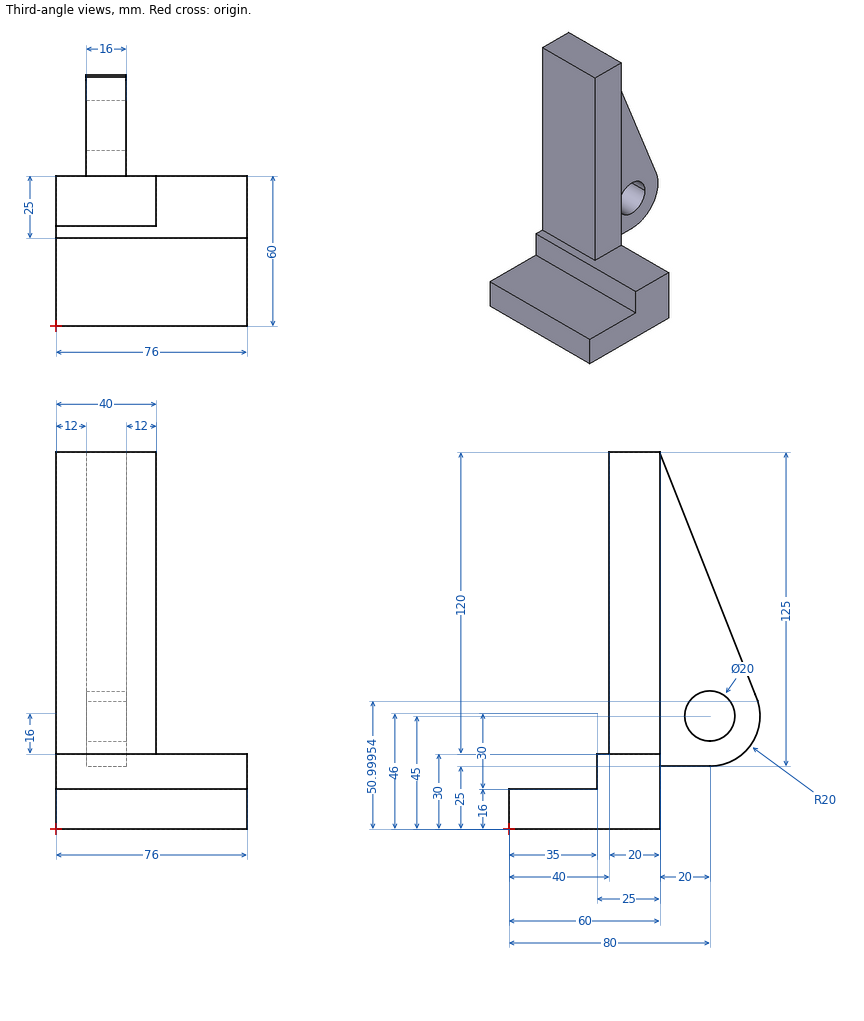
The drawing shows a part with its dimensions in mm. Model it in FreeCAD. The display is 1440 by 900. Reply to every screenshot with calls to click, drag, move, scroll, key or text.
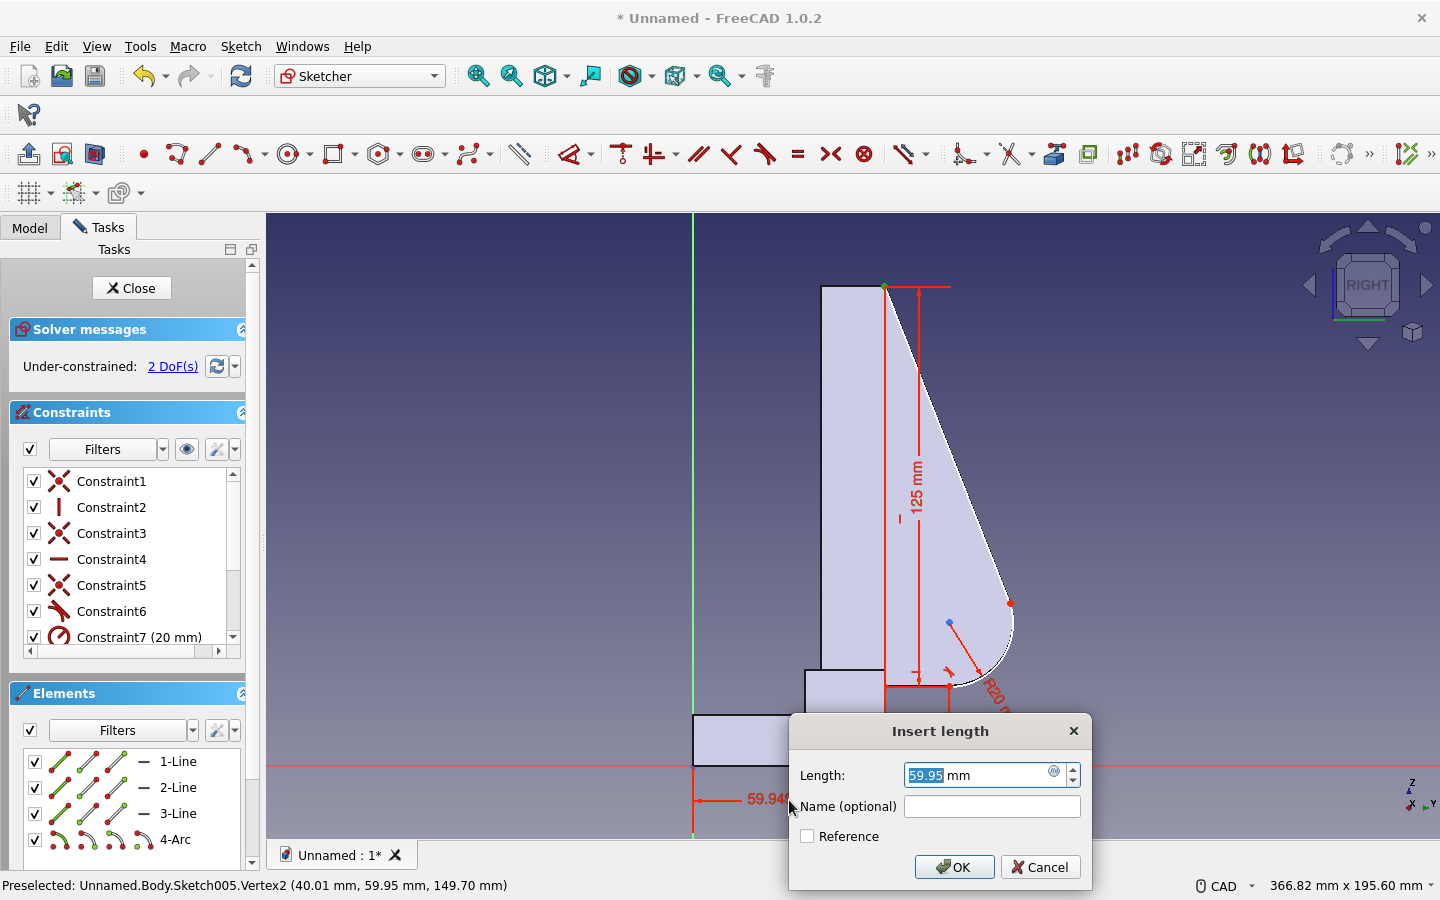
text(60)
key(Return)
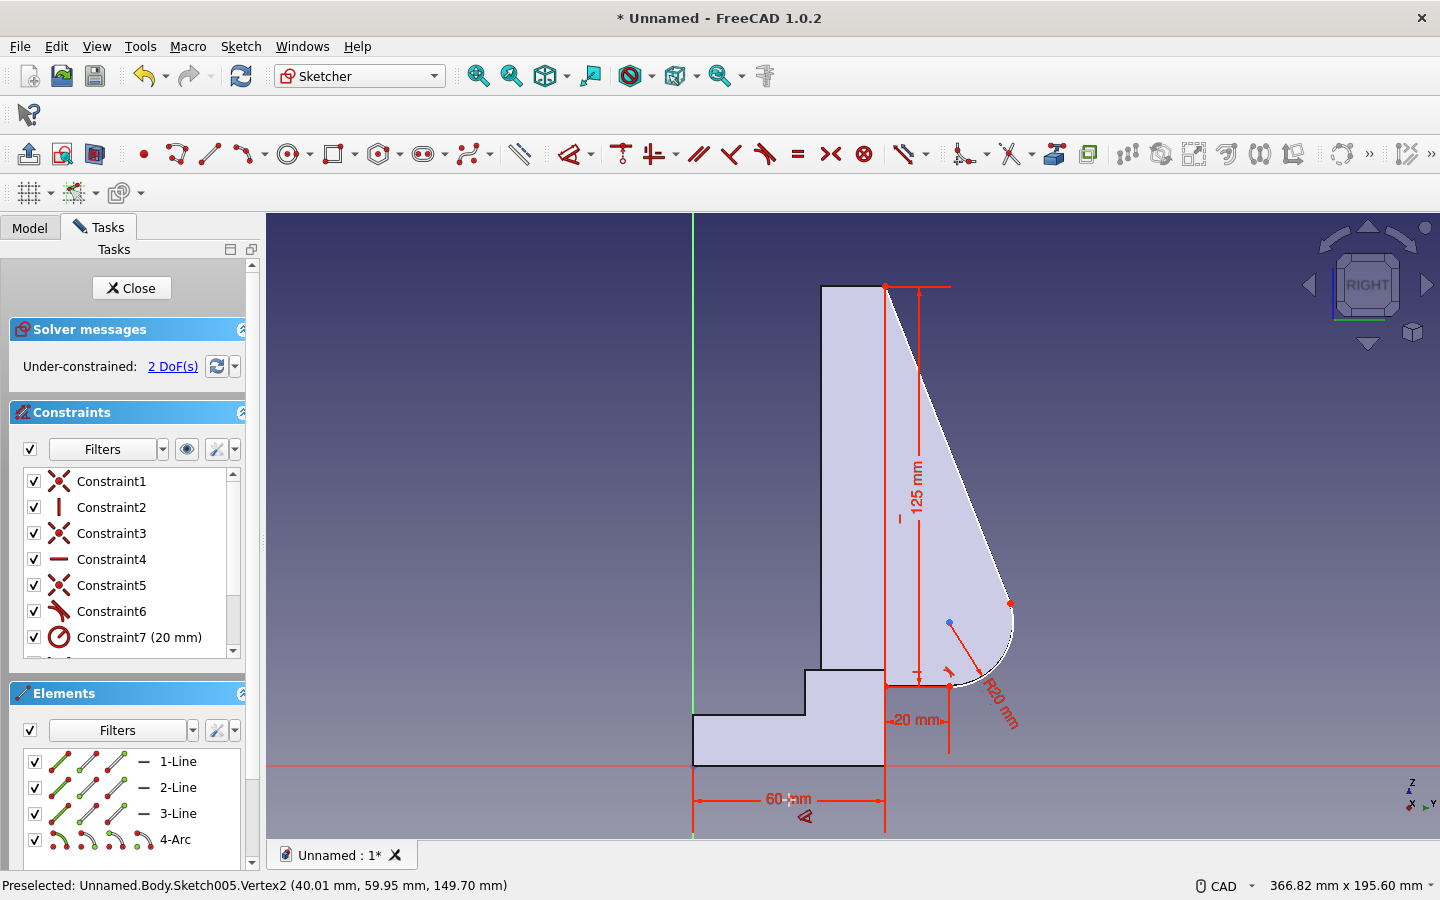
click(885, 687)
click(659, 727)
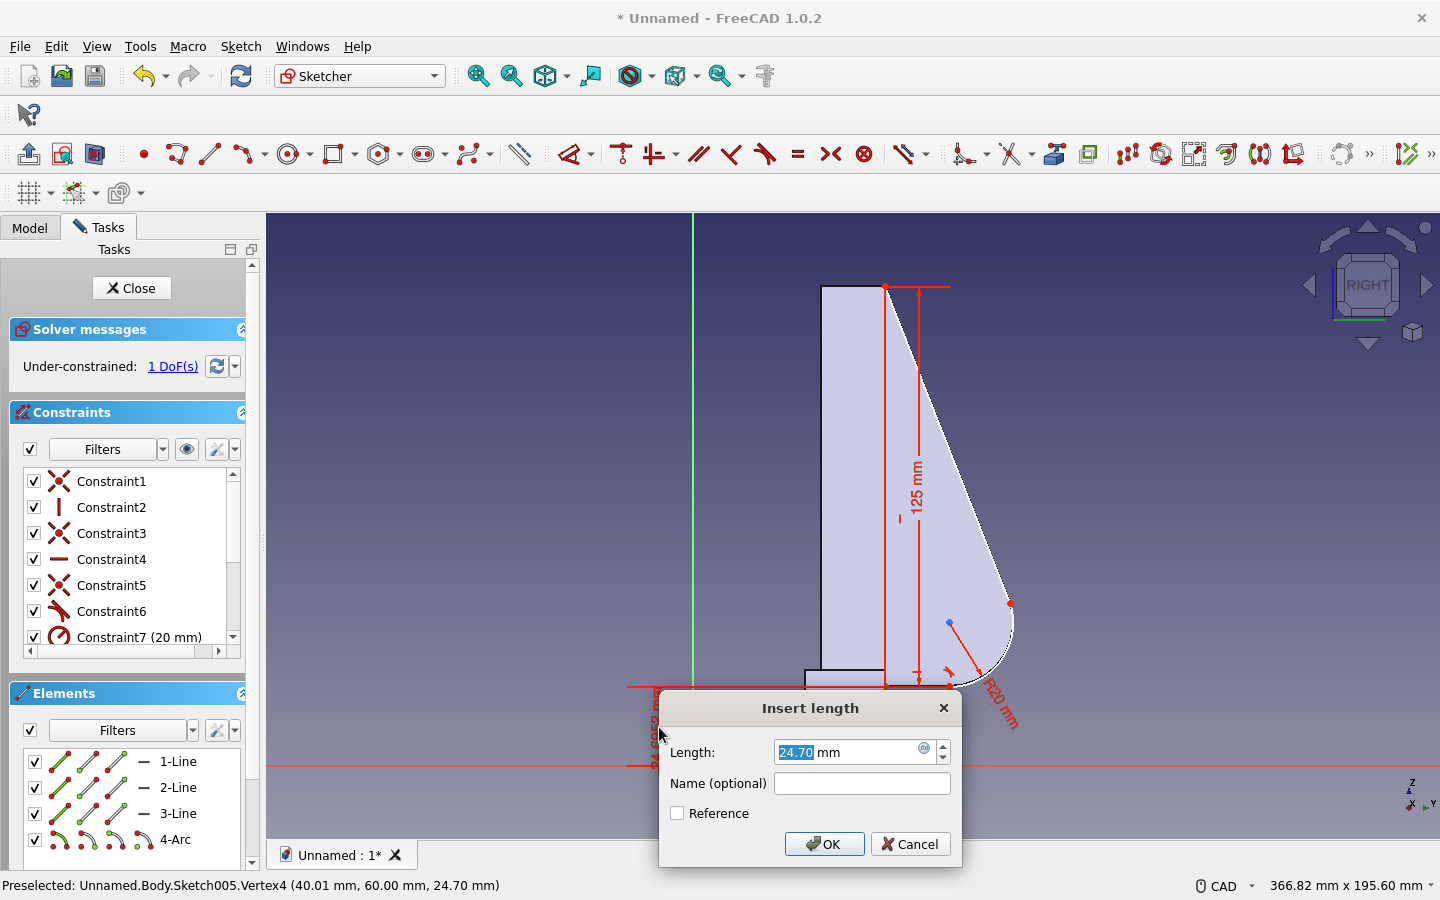
text(25)
key(Return)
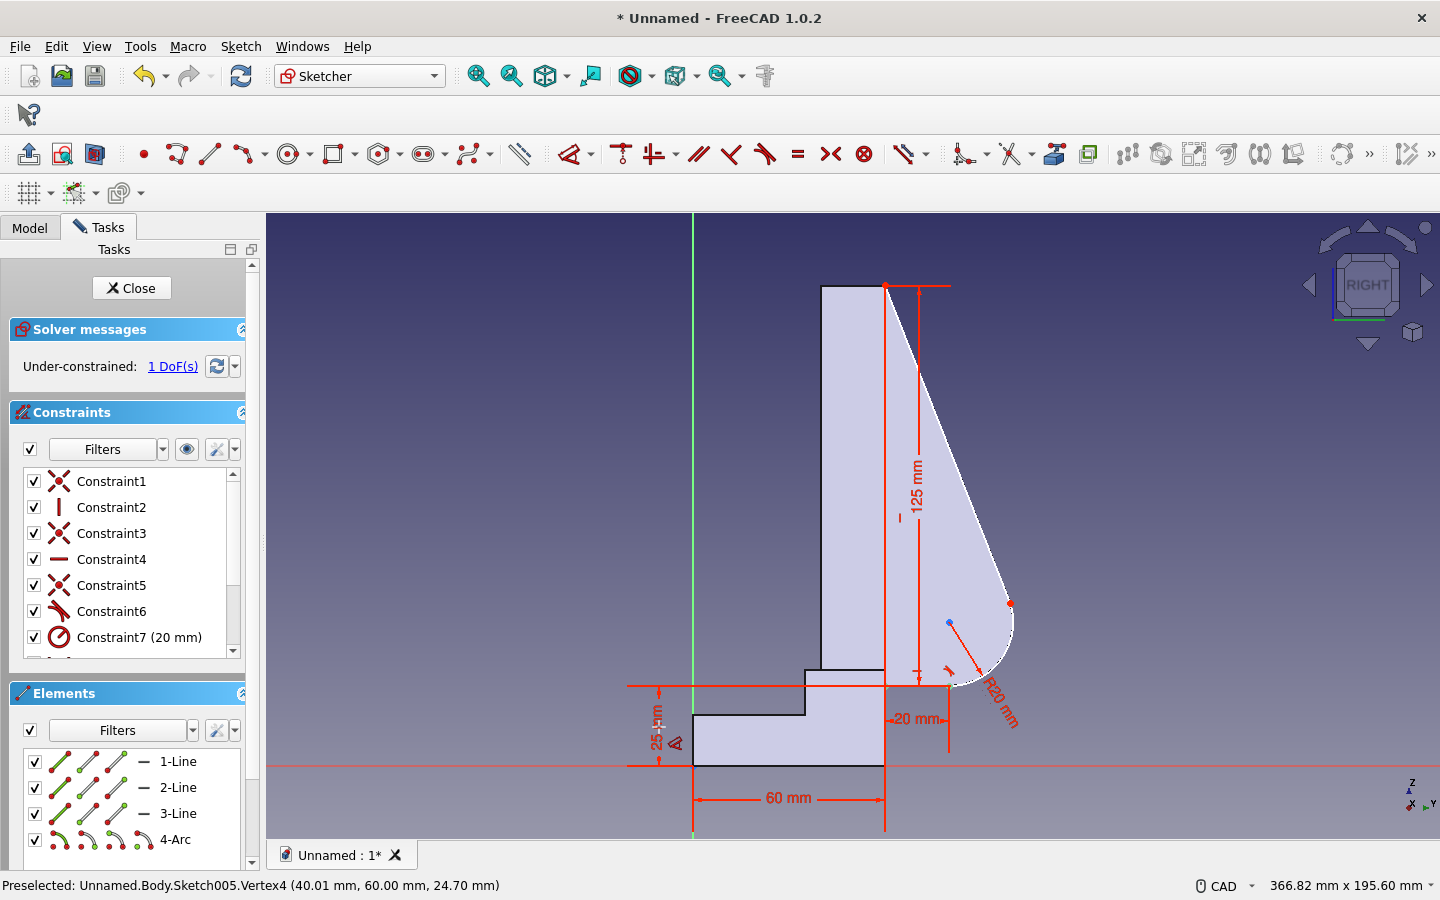
click(1011, 604)
click(1045, 648)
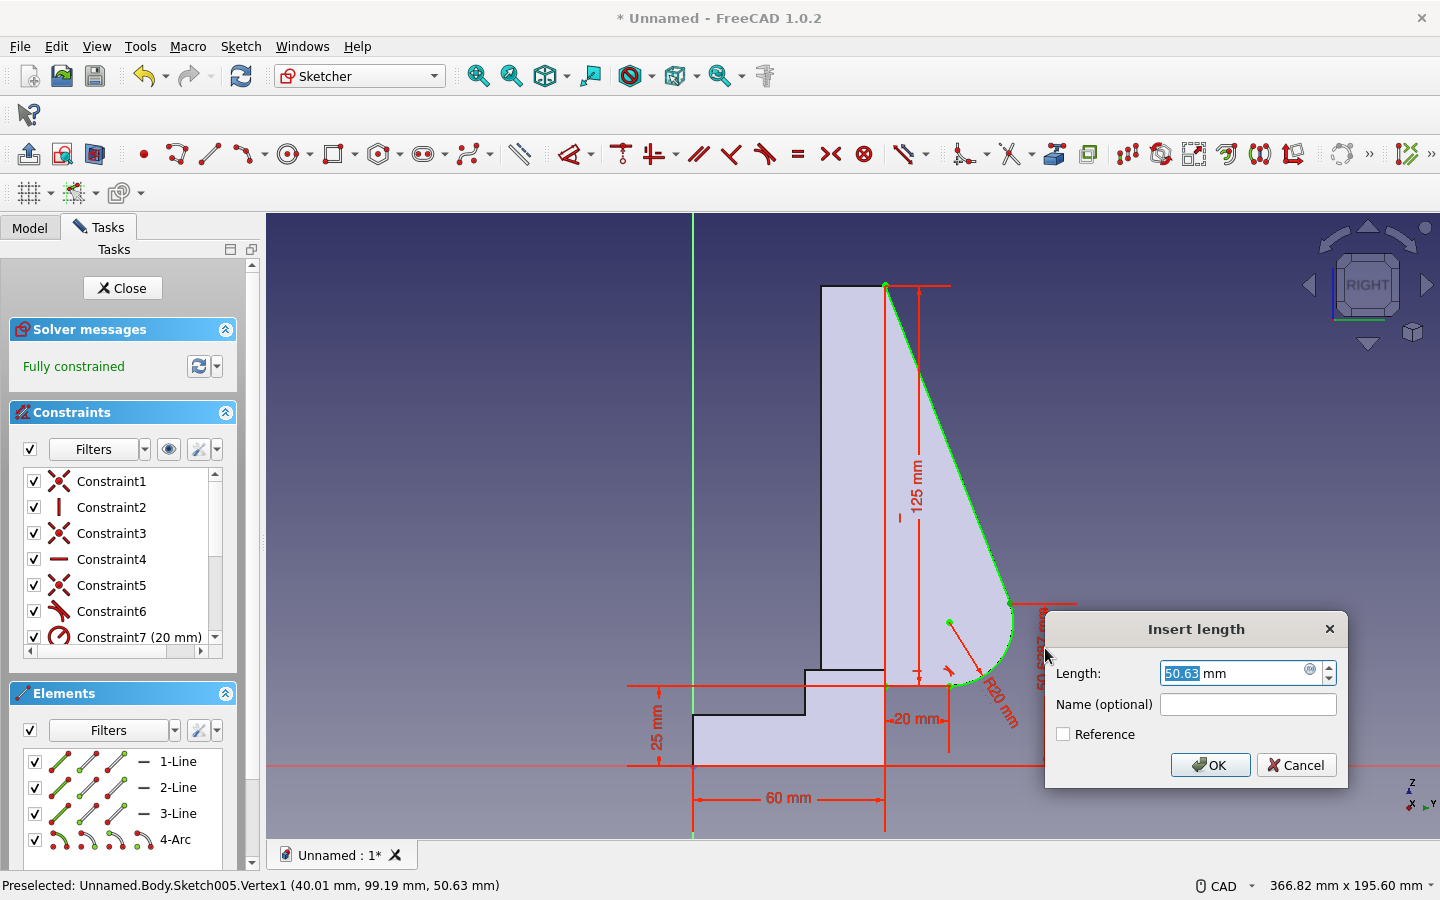
text(50.99954)
key(Return)
key(Escape)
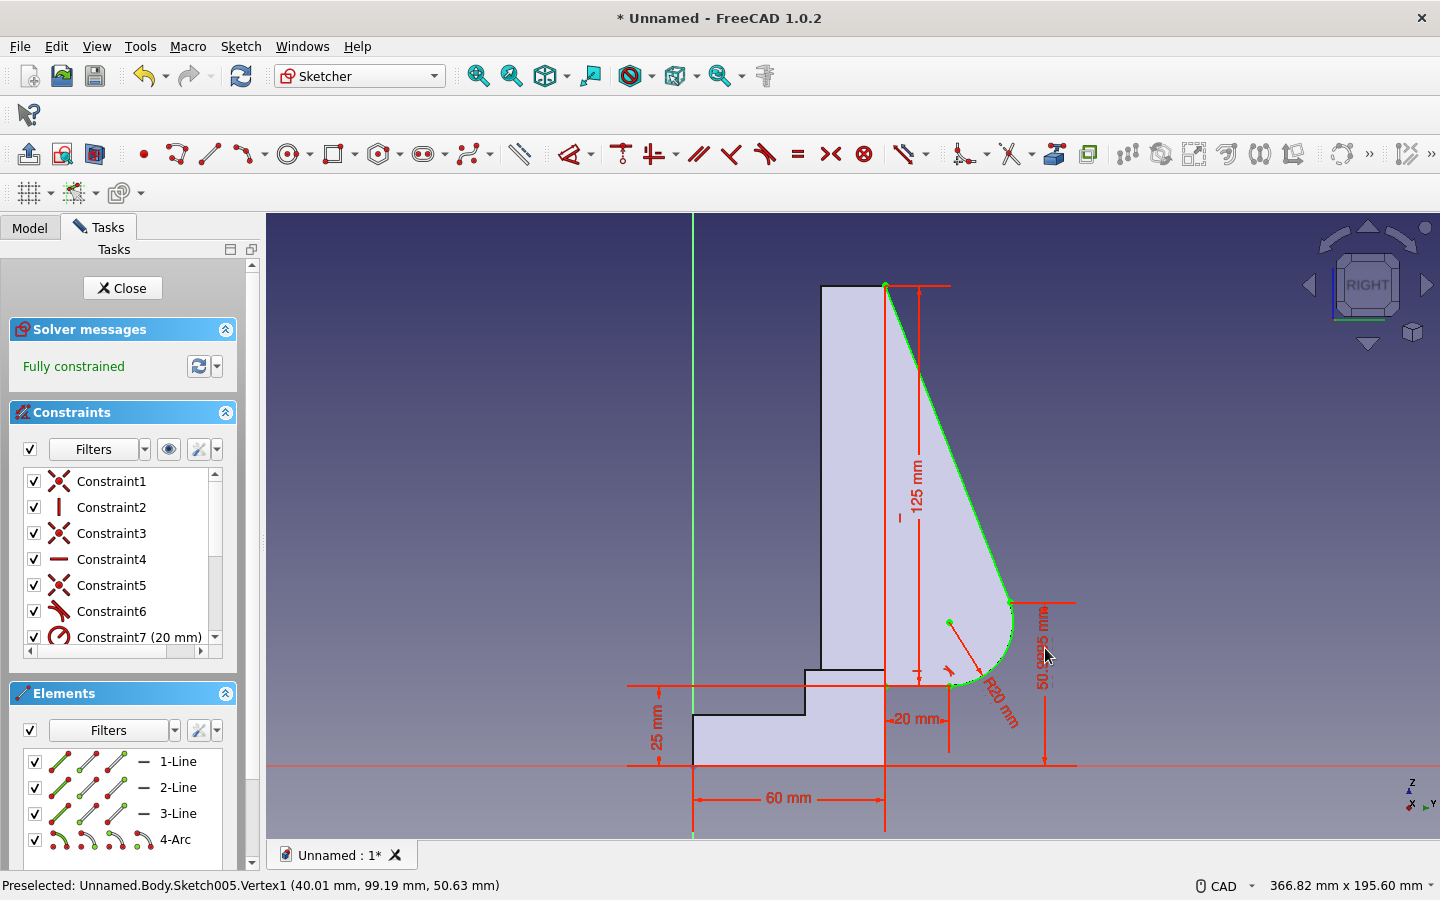
click(123, 288)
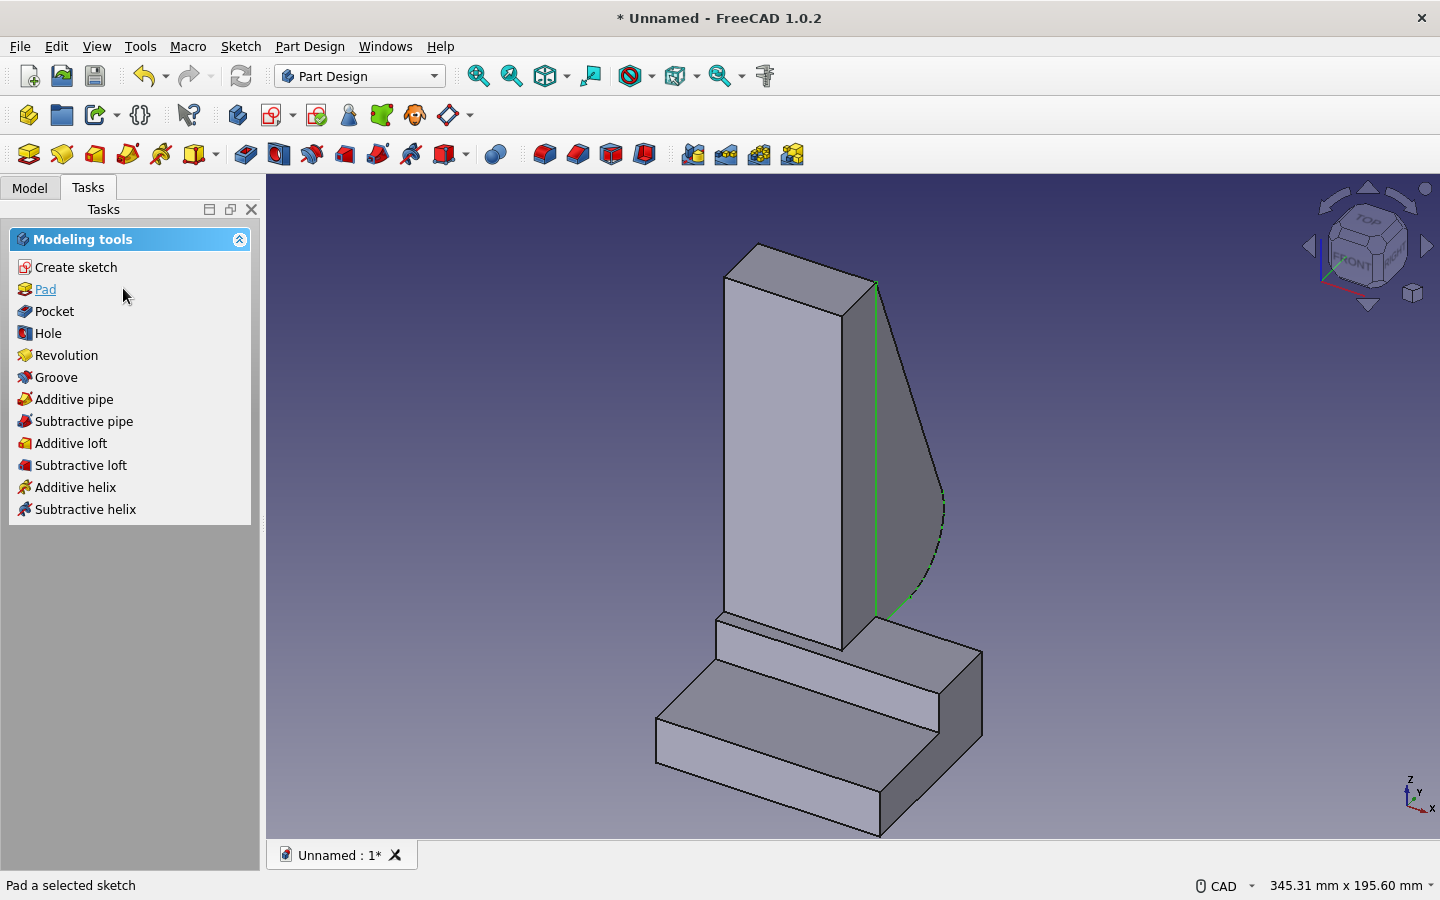
click(246, 154)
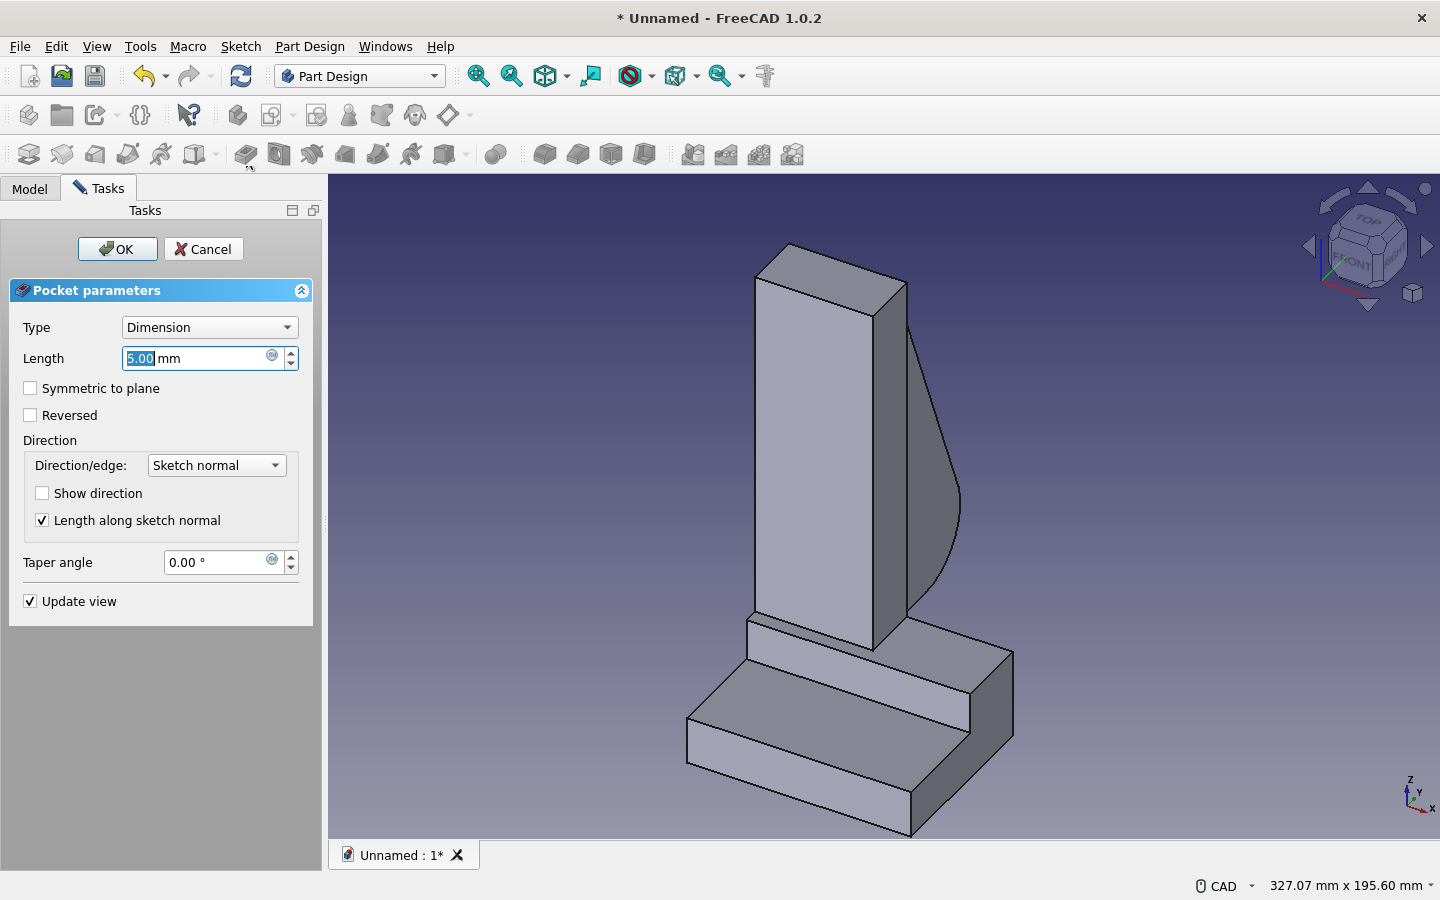
text(12)
key(Tab)